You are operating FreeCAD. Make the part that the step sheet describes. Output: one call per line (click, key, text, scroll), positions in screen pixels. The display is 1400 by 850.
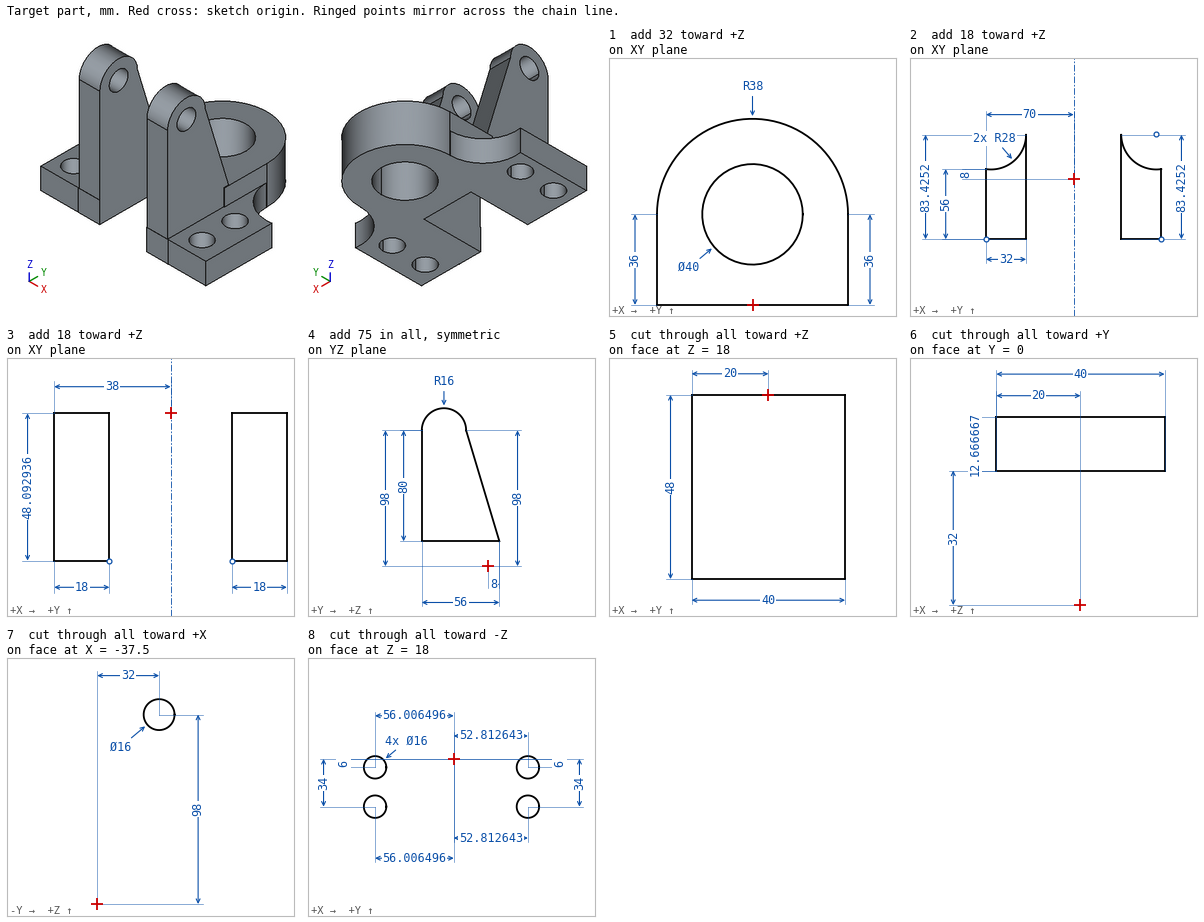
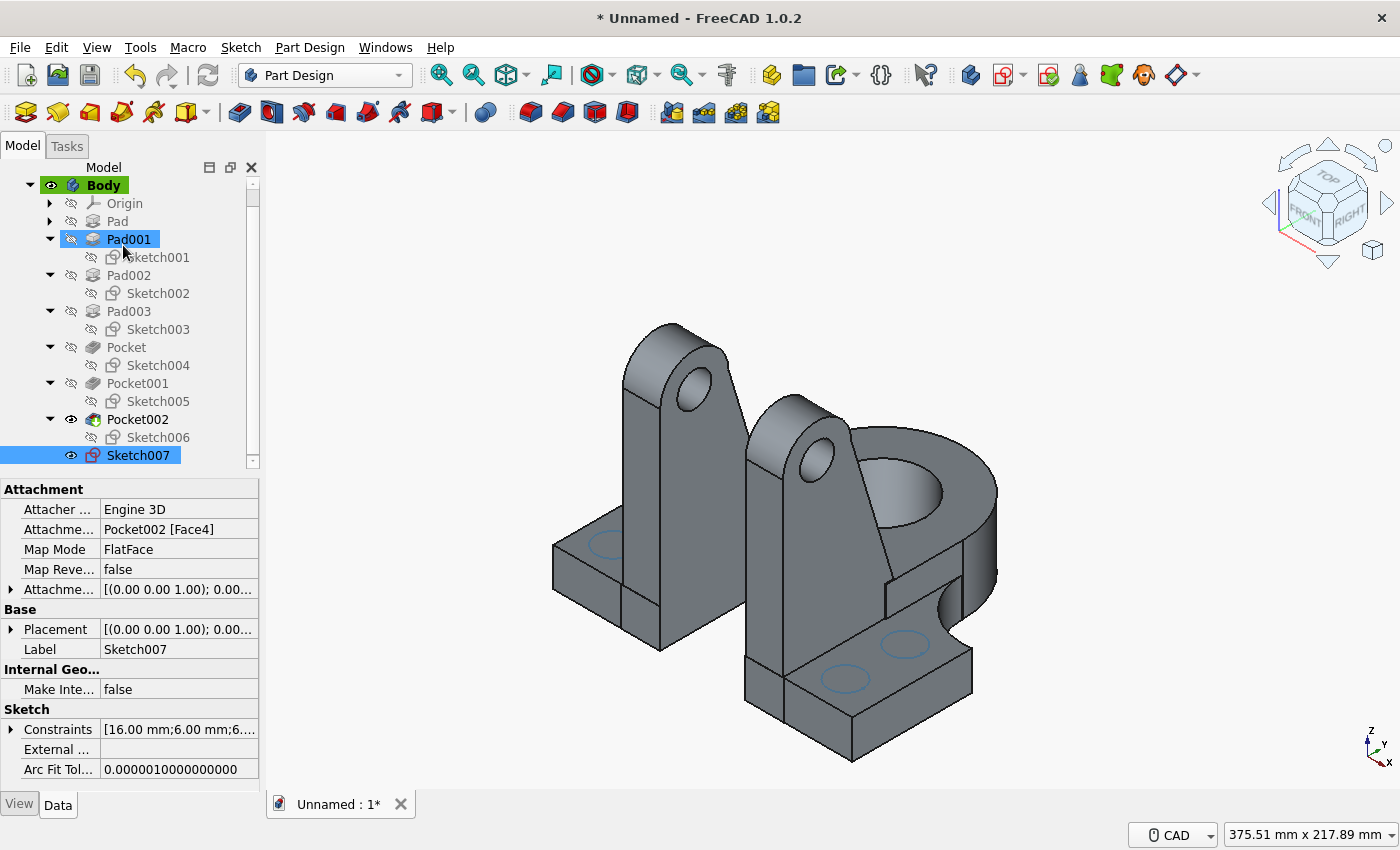
click(240, 112)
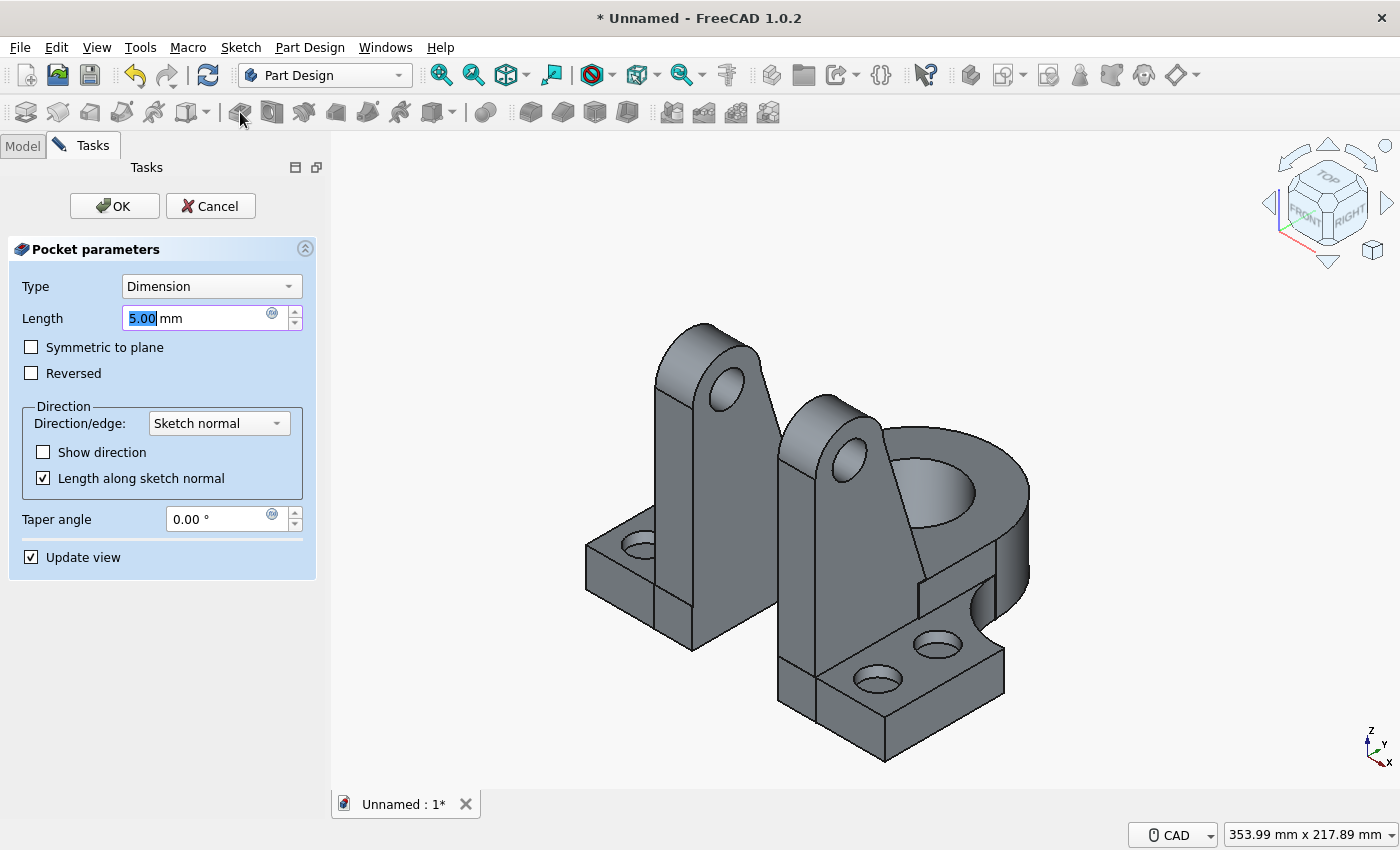
click(212, 286)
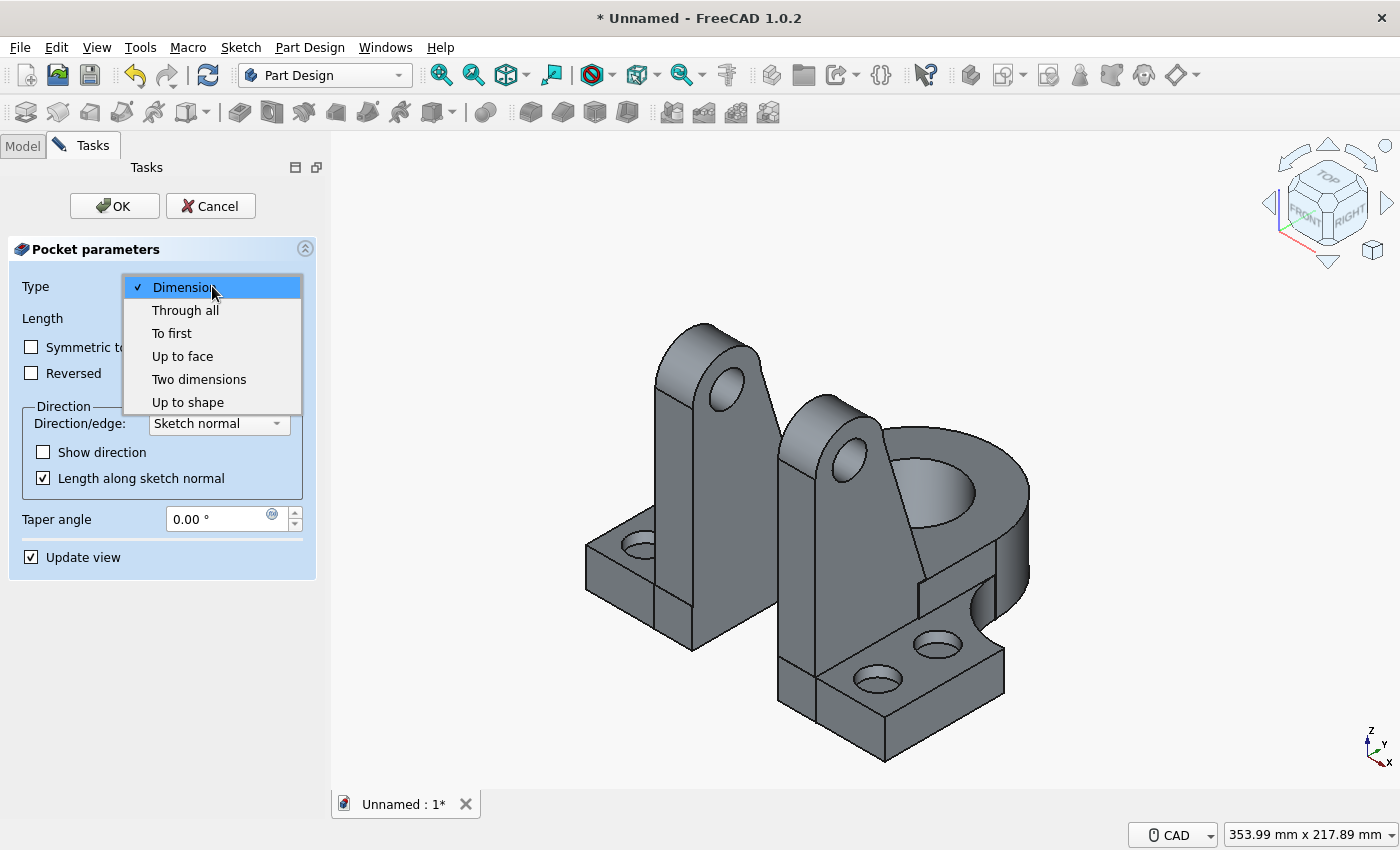
click(212, 310)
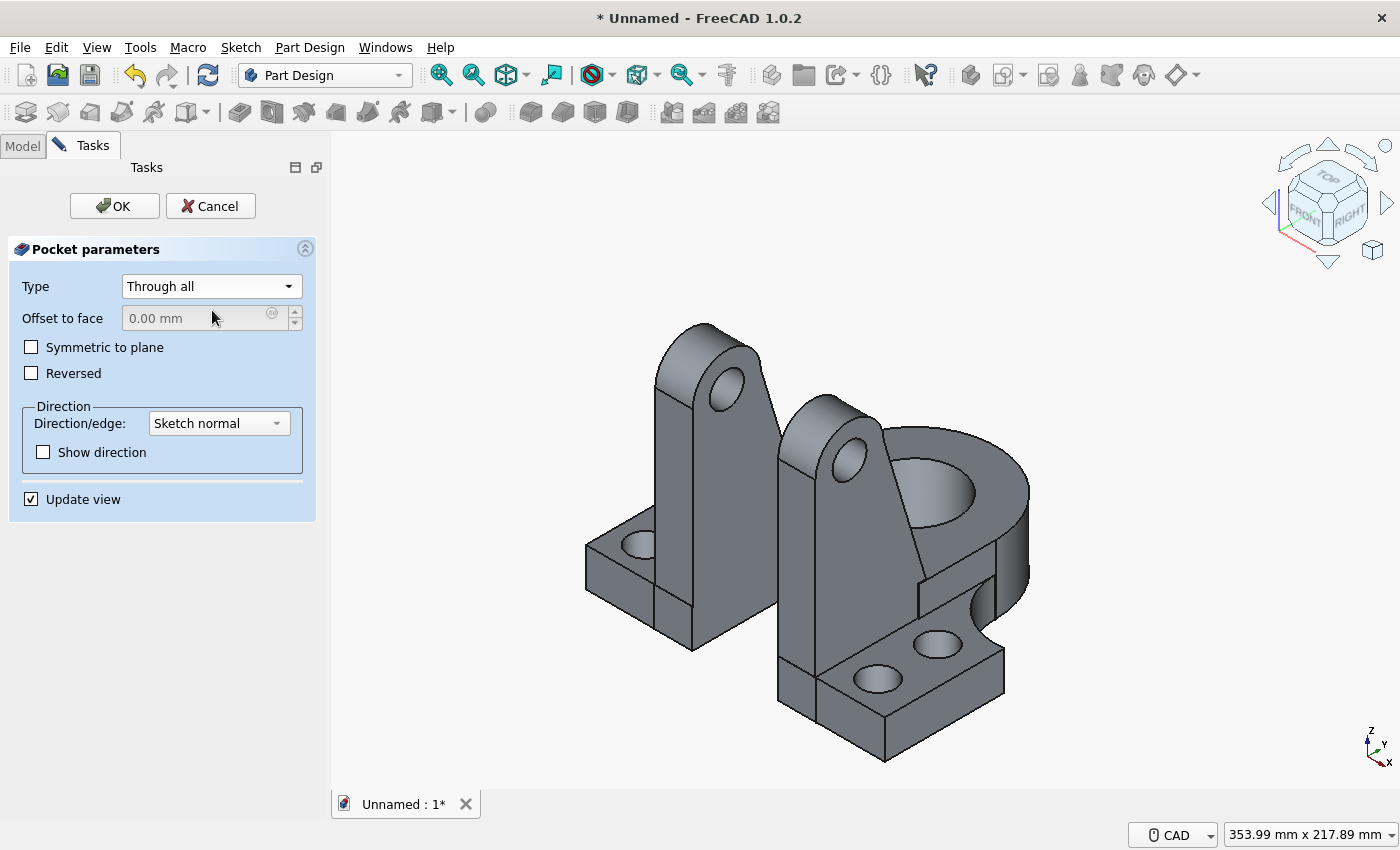
click(115, 206)